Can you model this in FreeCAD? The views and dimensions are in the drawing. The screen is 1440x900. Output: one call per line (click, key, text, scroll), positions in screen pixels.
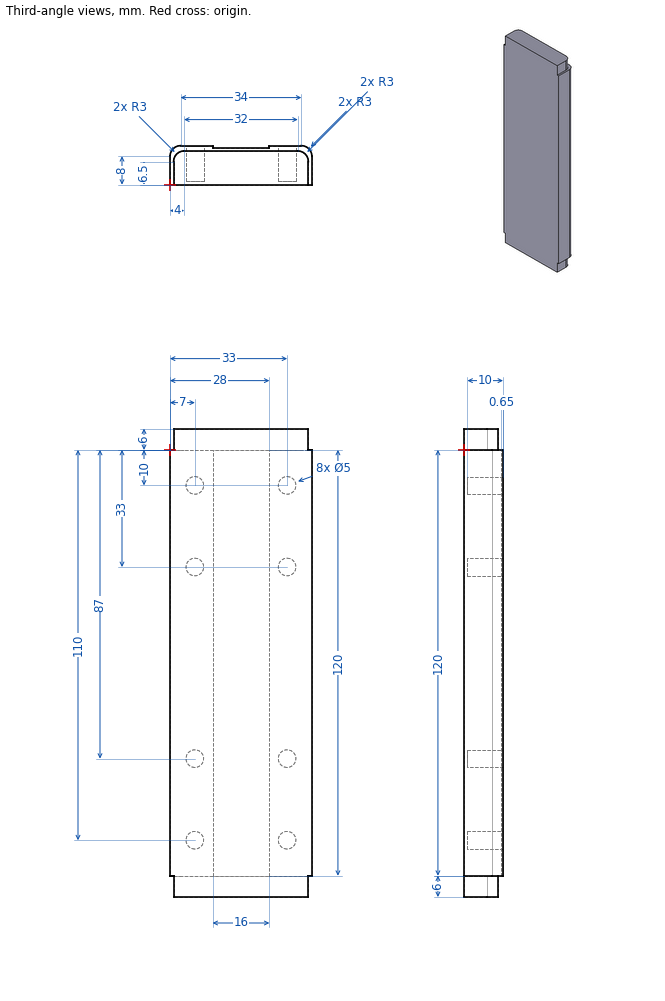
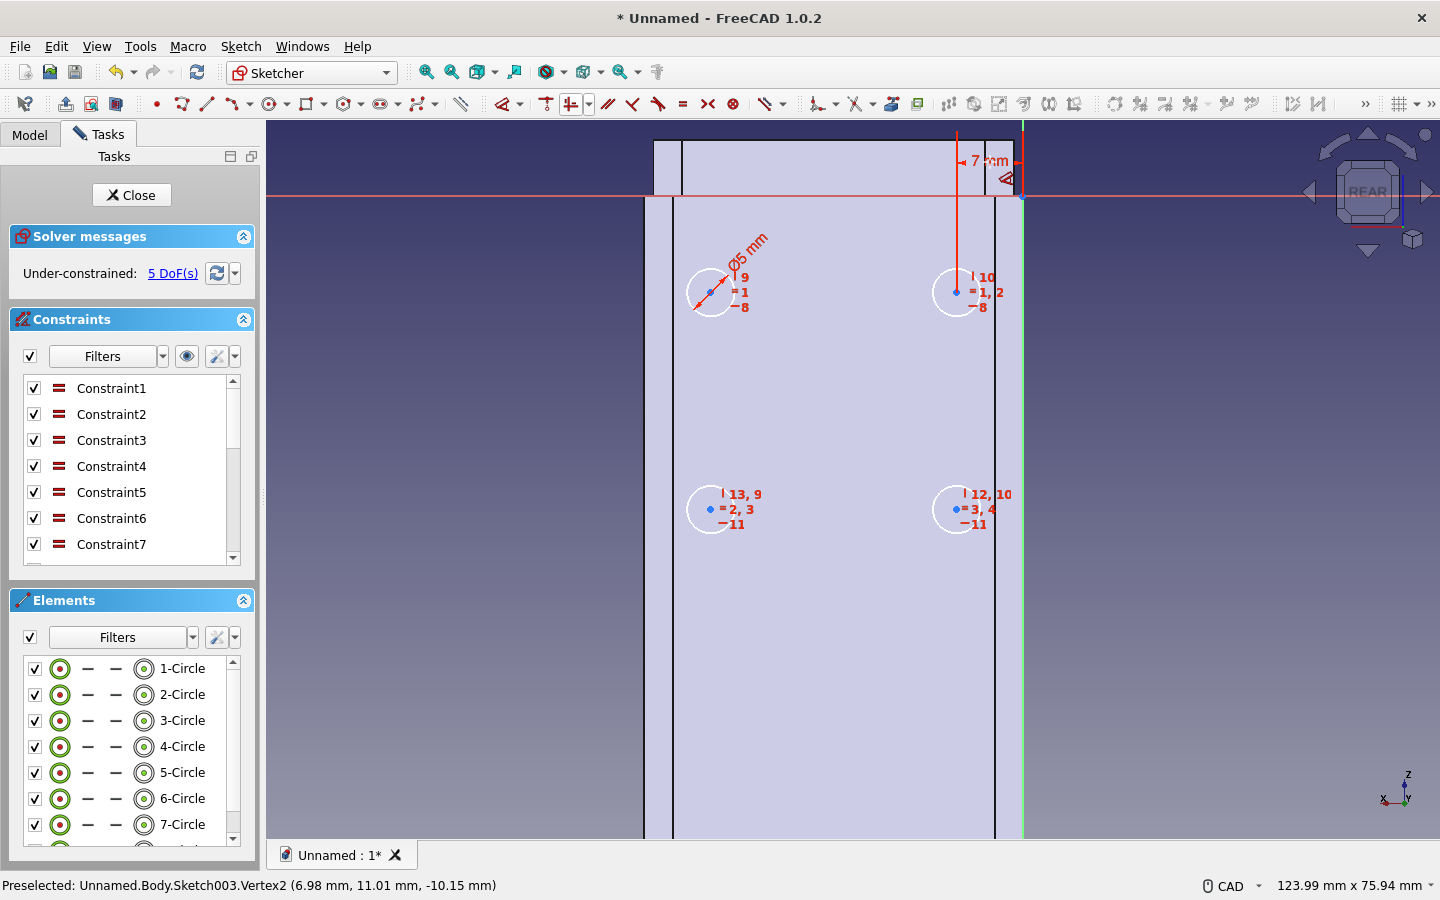
click(711, 293)
click(867, 162)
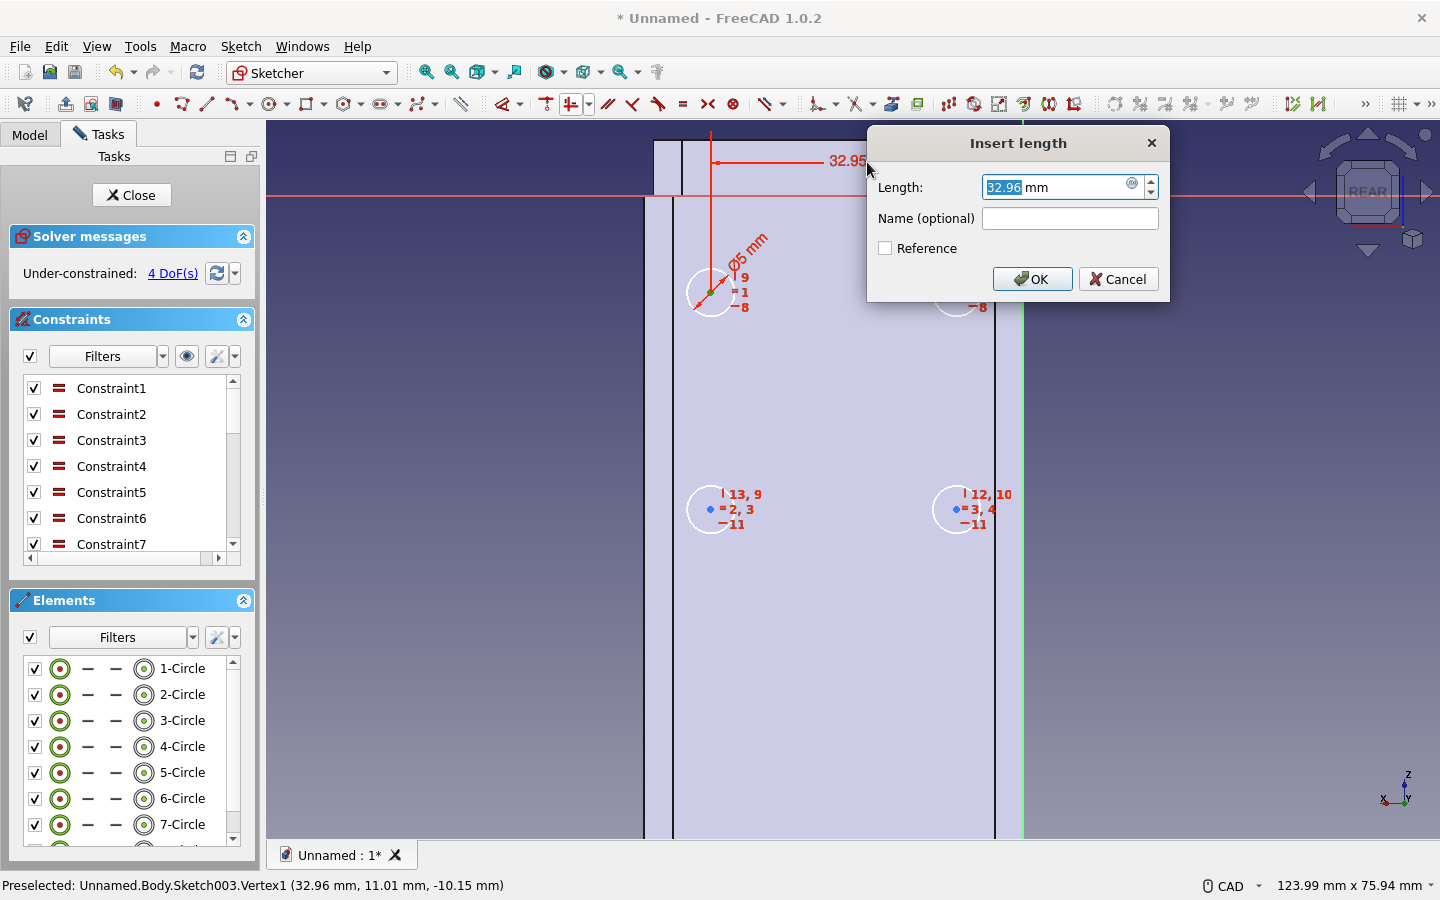
text(33)
key(Return)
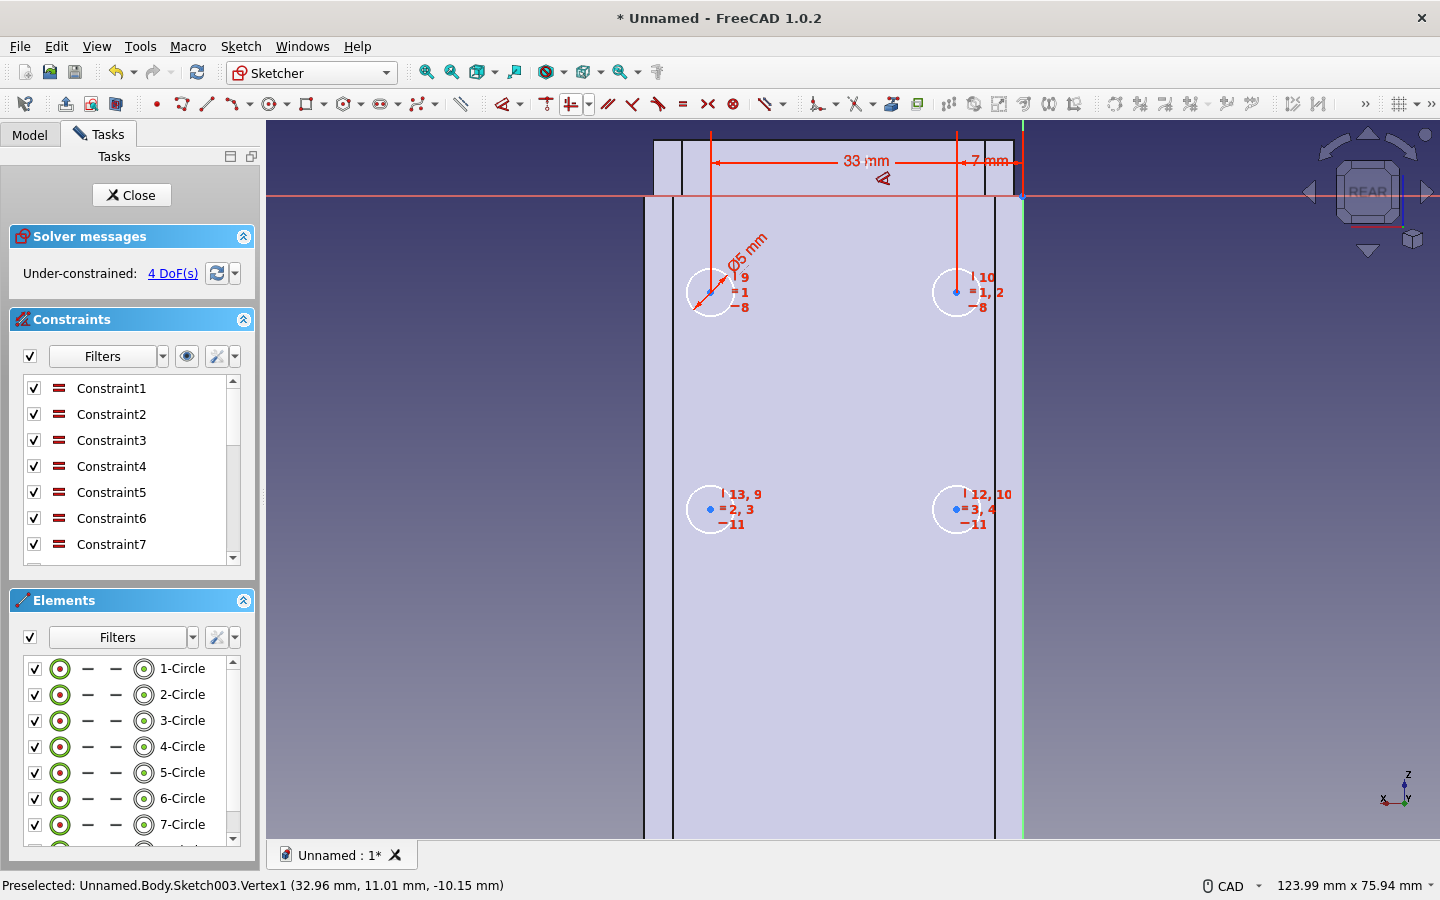
click(711, 293)
click(1057, 245)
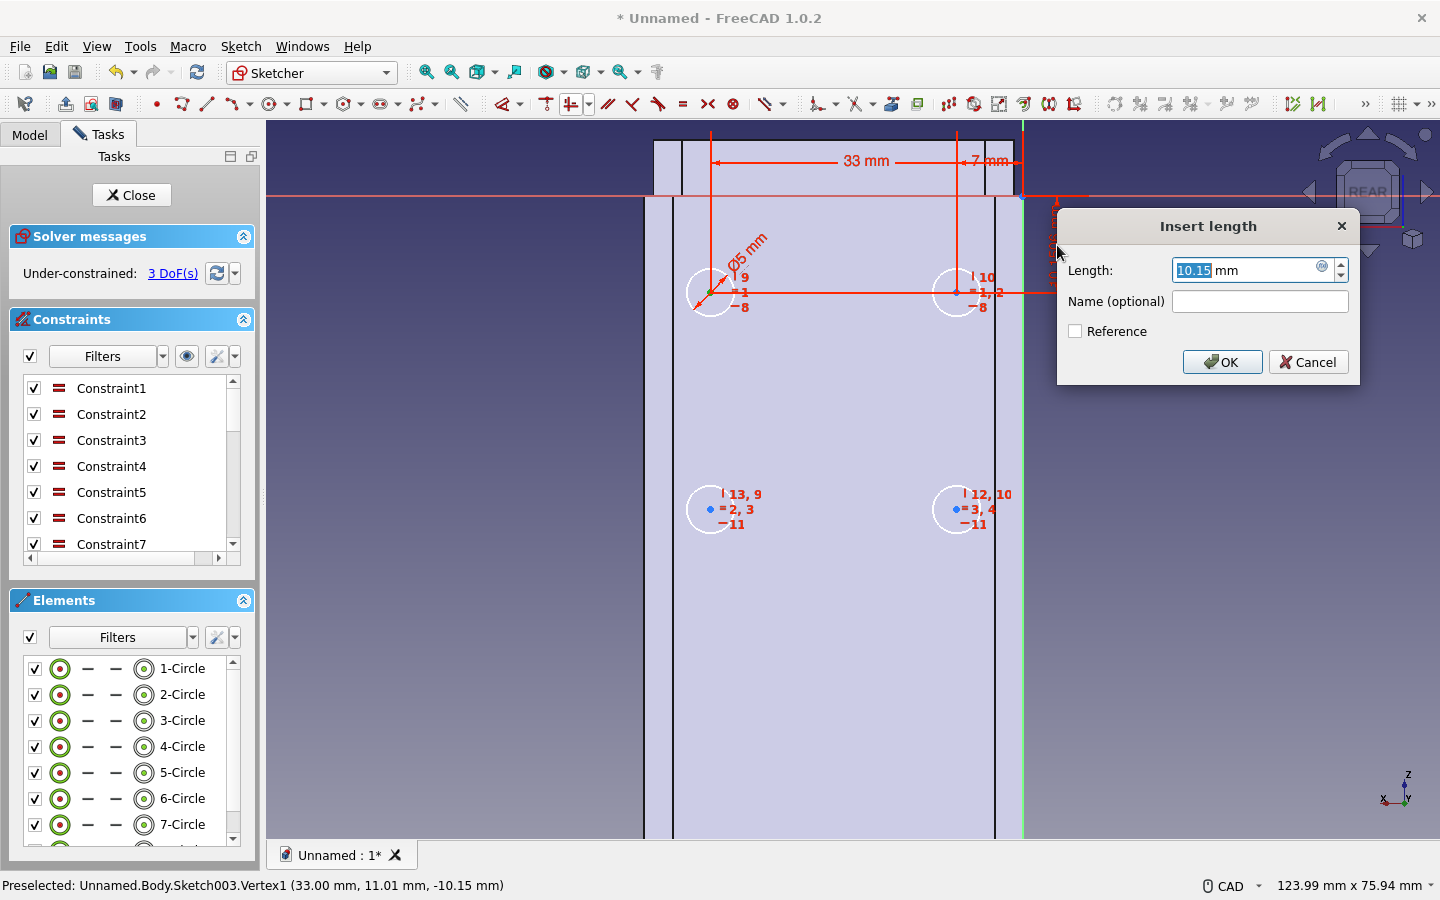
text(10)
key(Return)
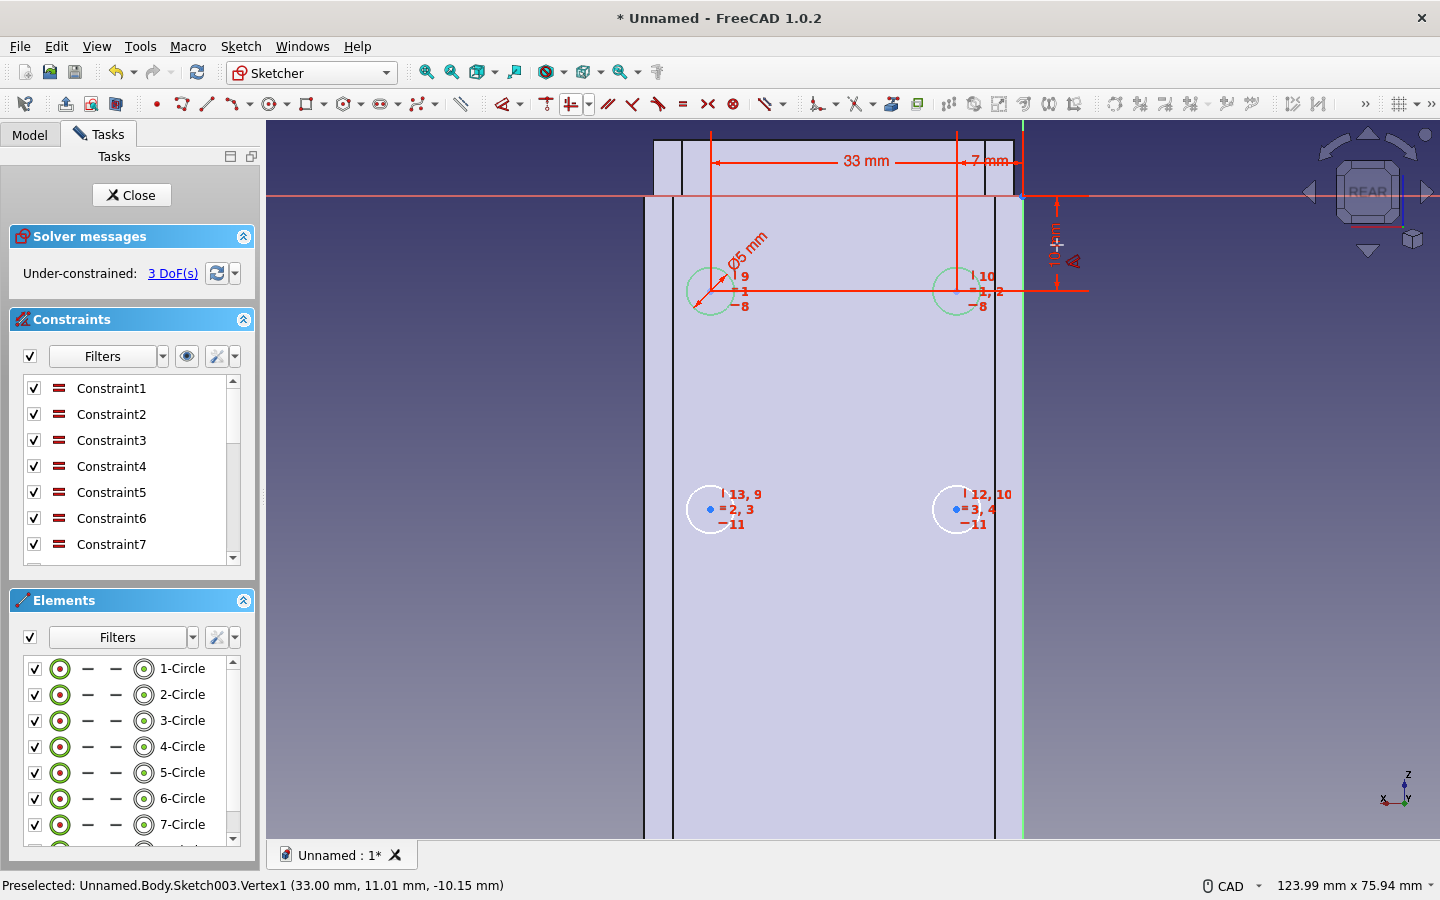
click(711, 510)
click(1057, 353)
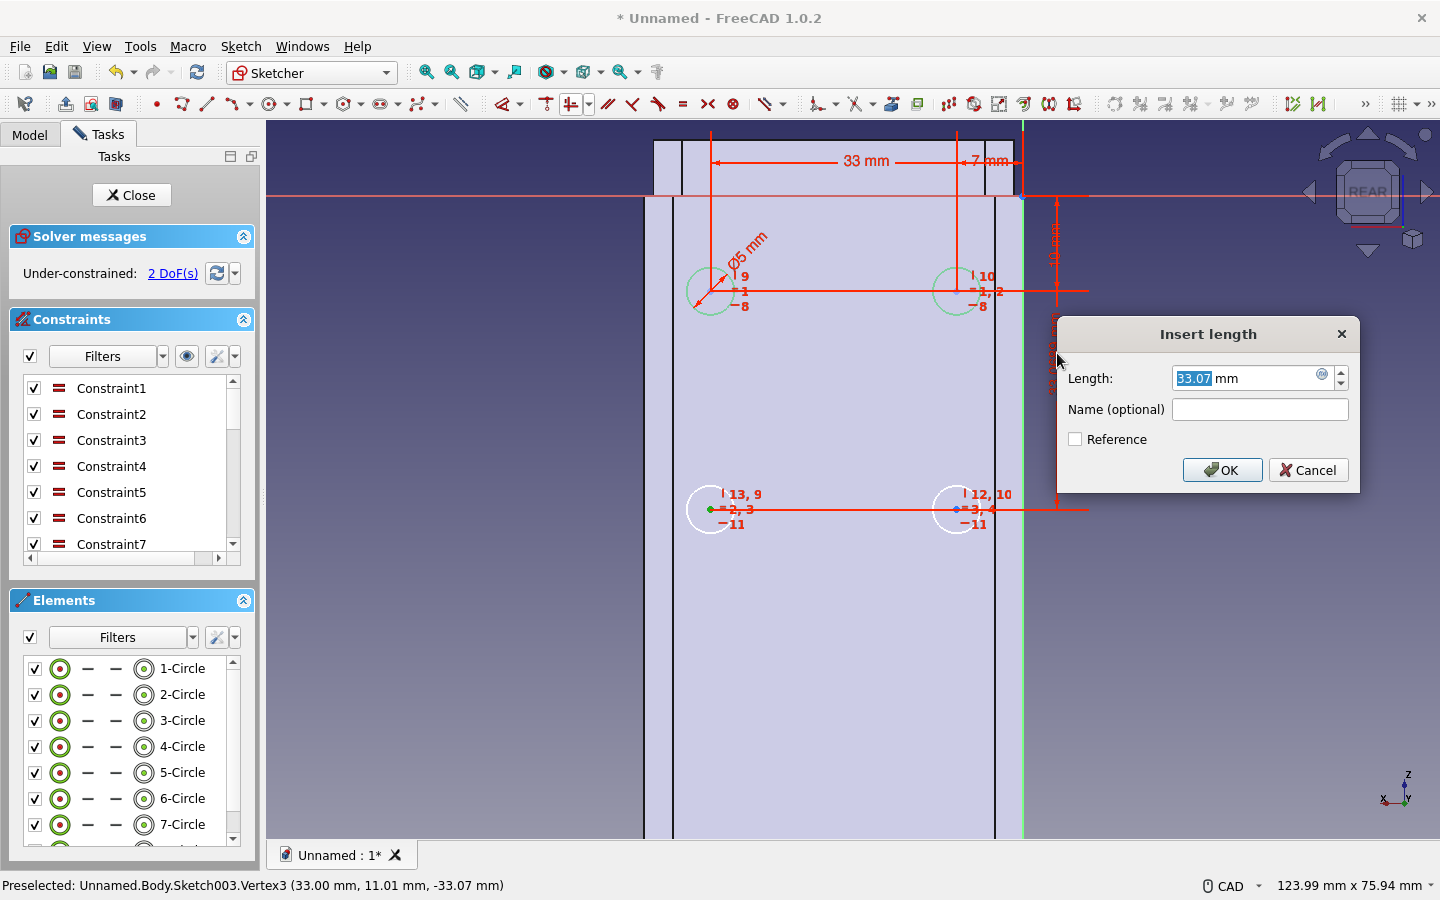
text(33)
key(Return)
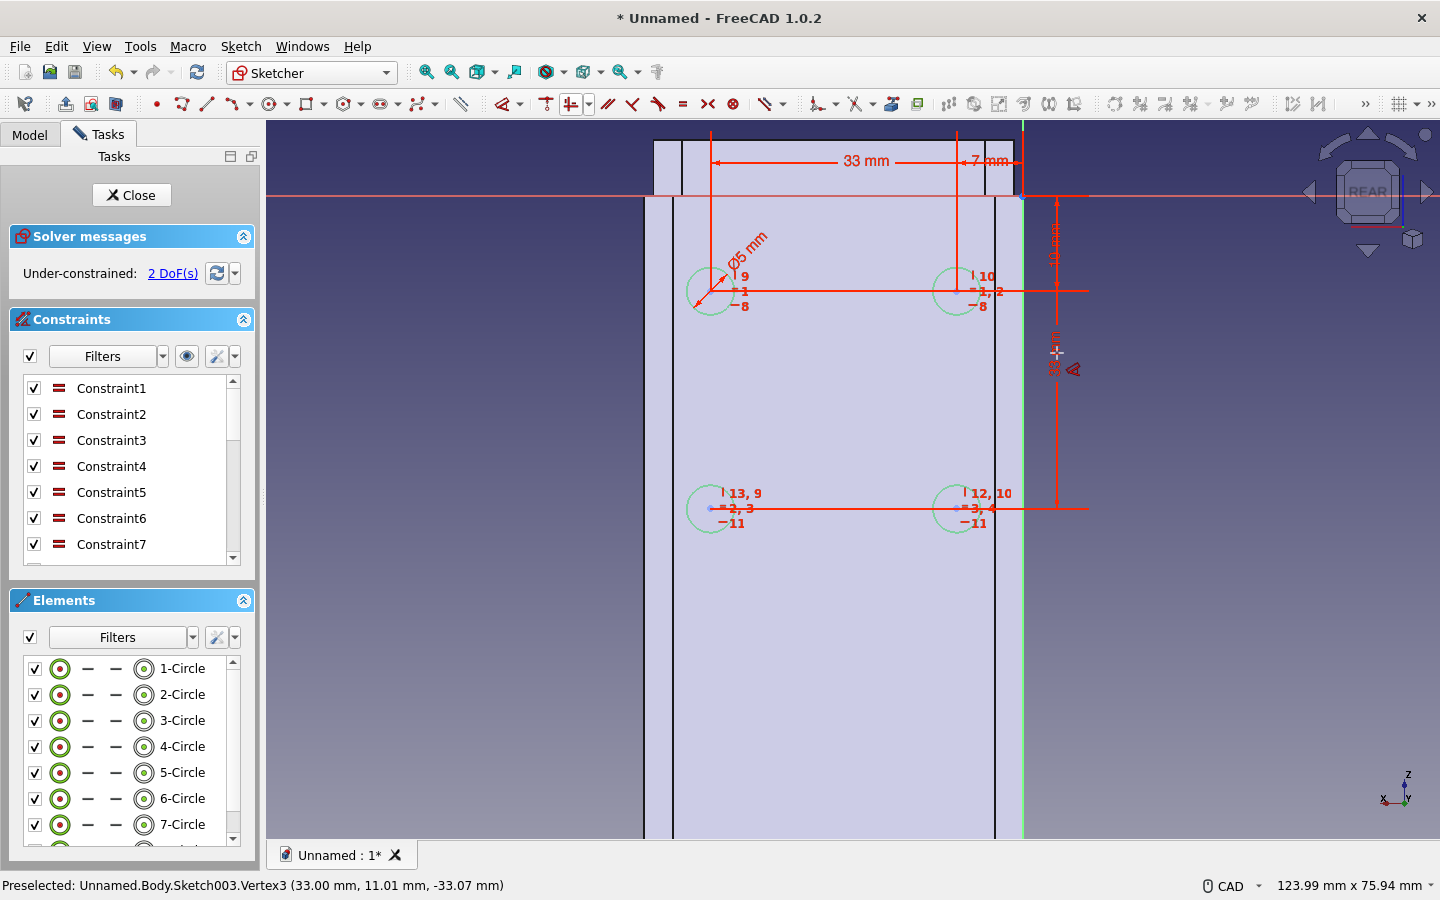
scroll(727, 276, down, 4)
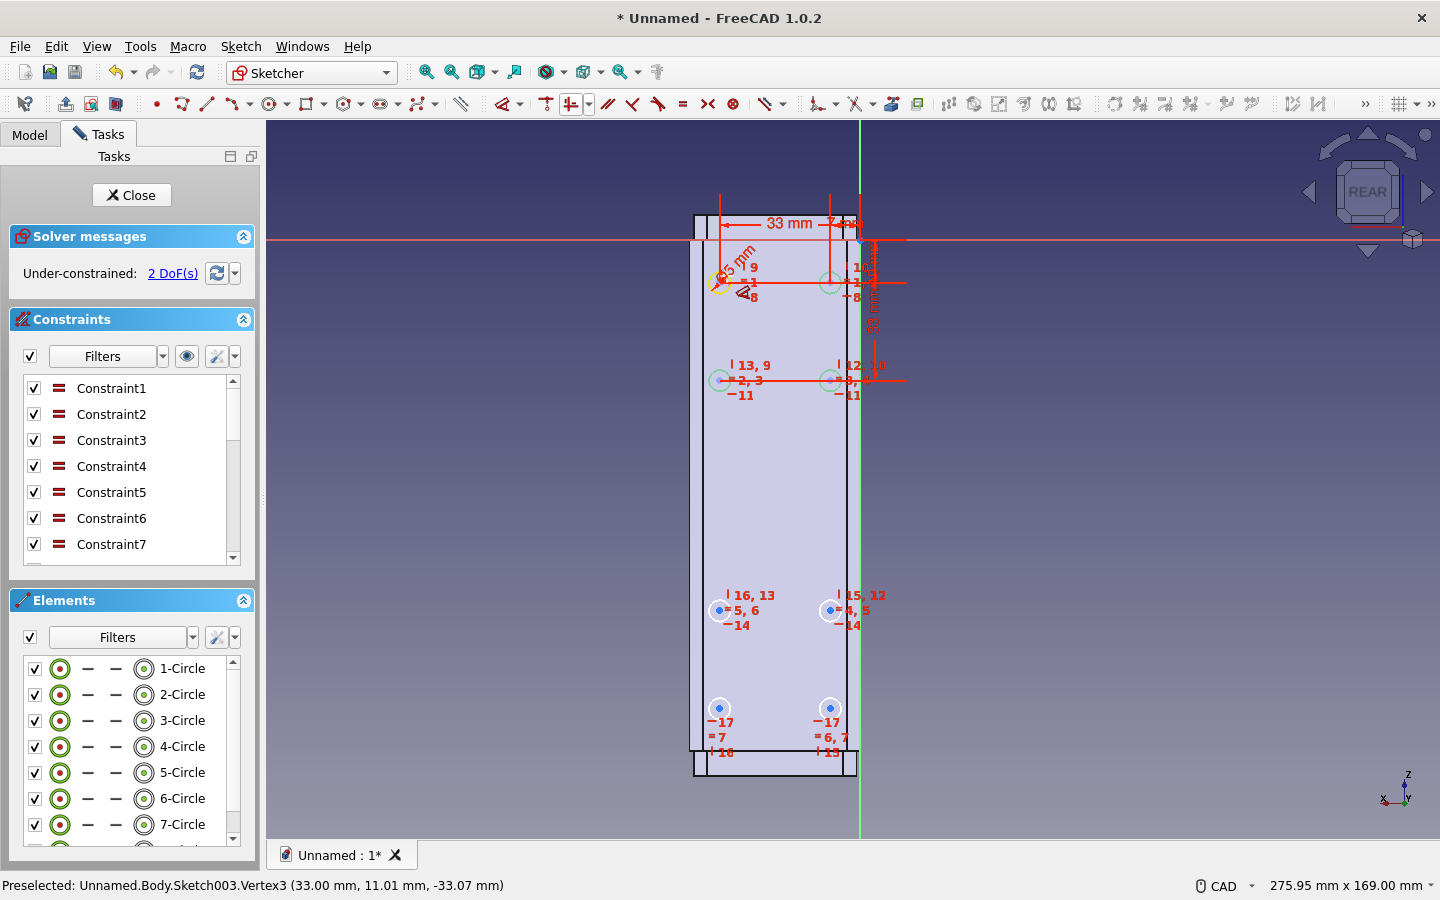
click(830, 611)
click(894, 426)